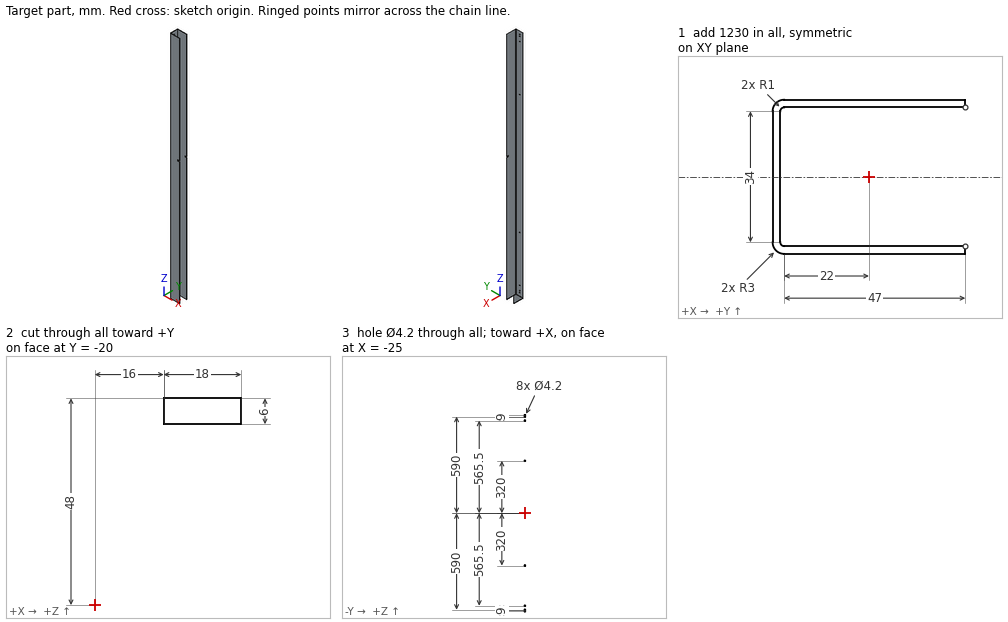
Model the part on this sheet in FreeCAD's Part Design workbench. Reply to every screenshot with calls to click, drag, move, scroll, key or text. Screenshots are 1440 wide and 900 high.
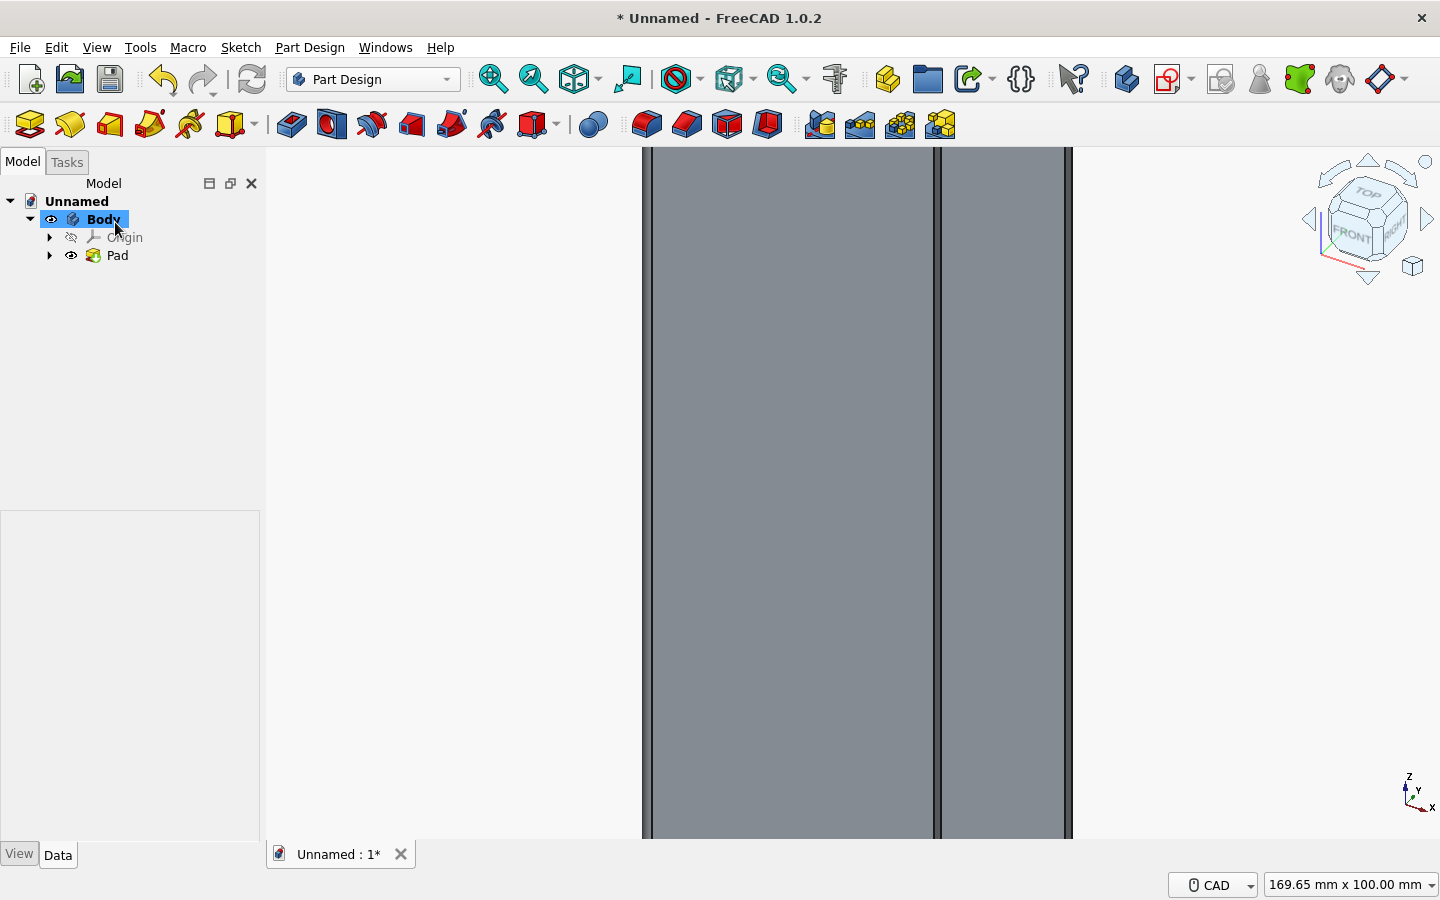
key(v)
key(f)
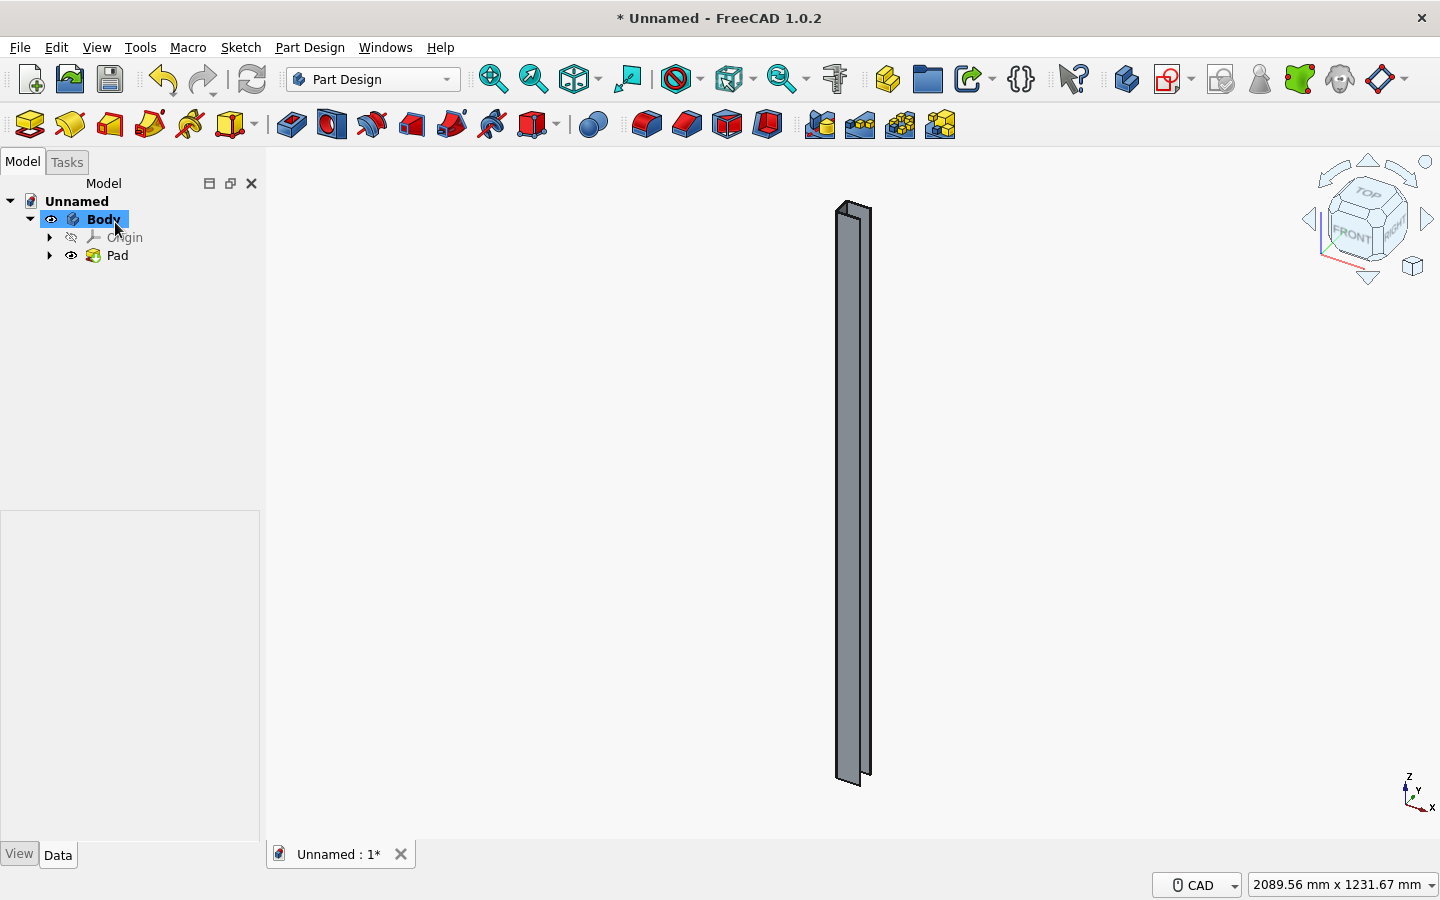
click(848, 255)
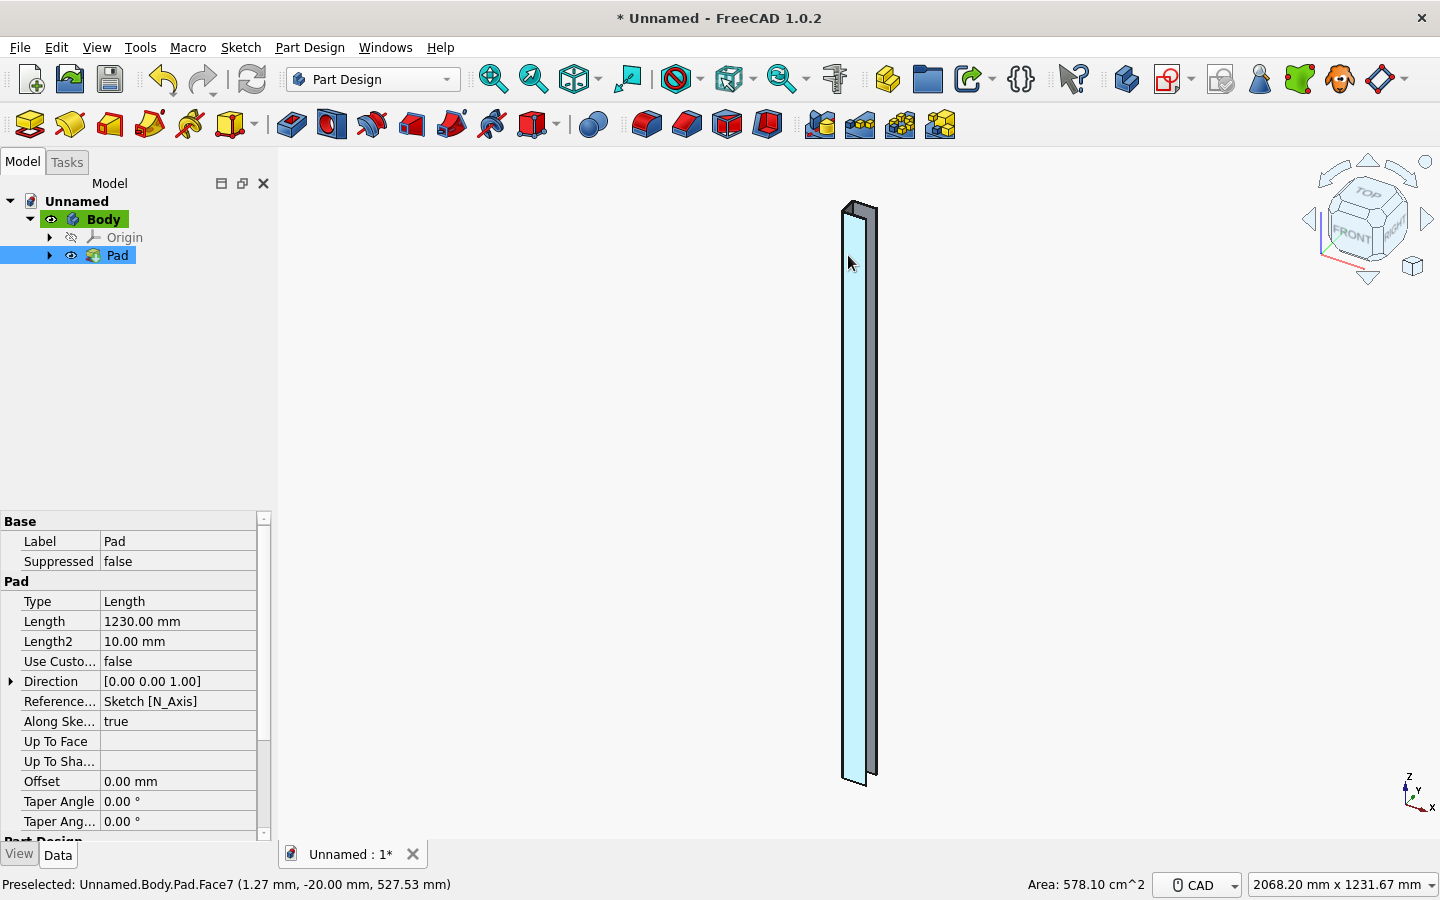
click(1168, 80)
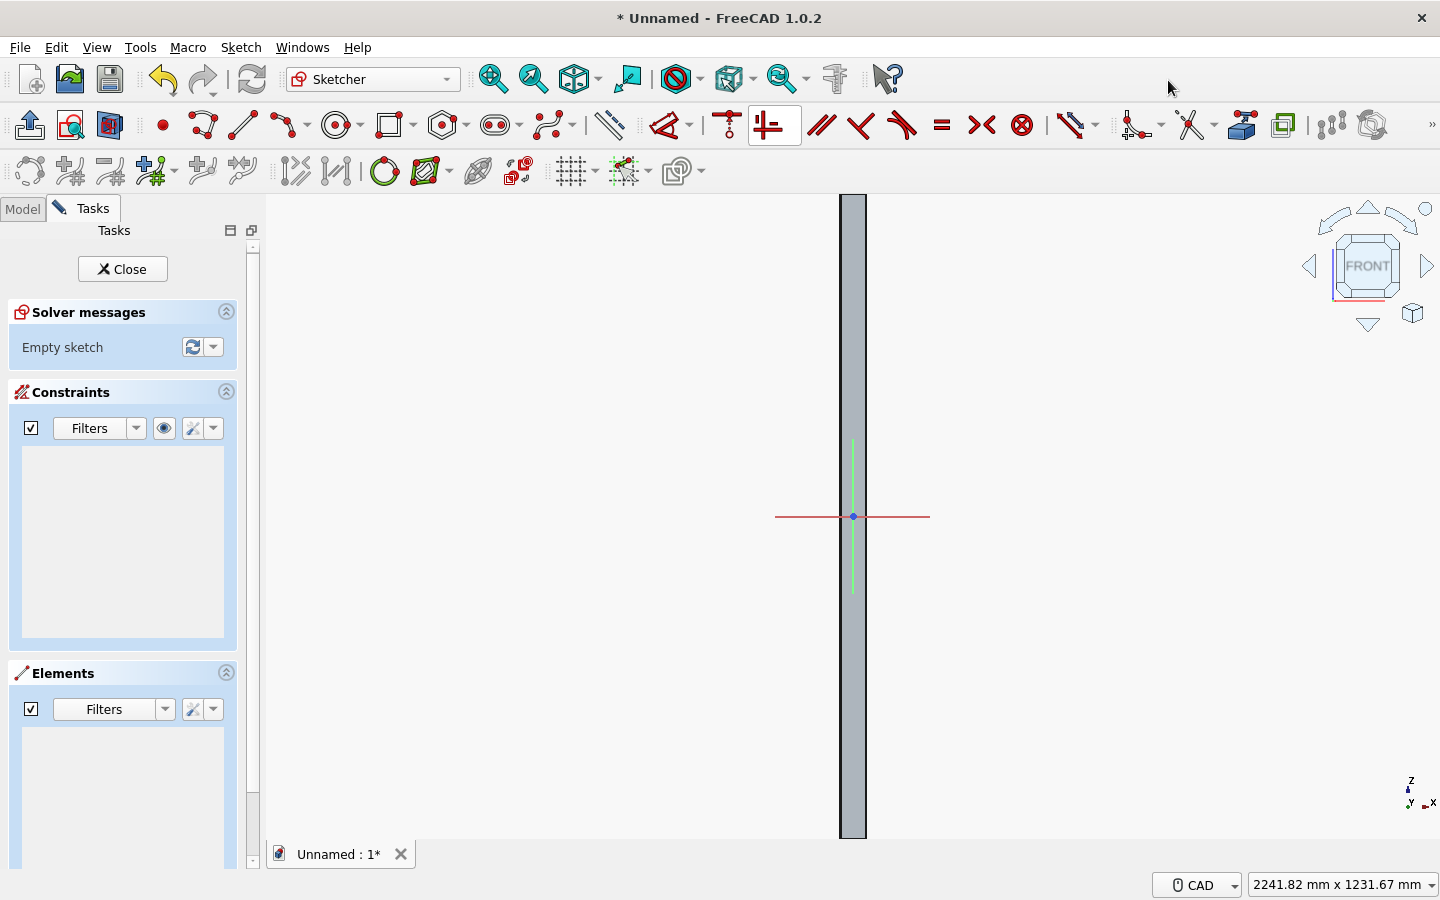
scroll(870, 492, up, 15)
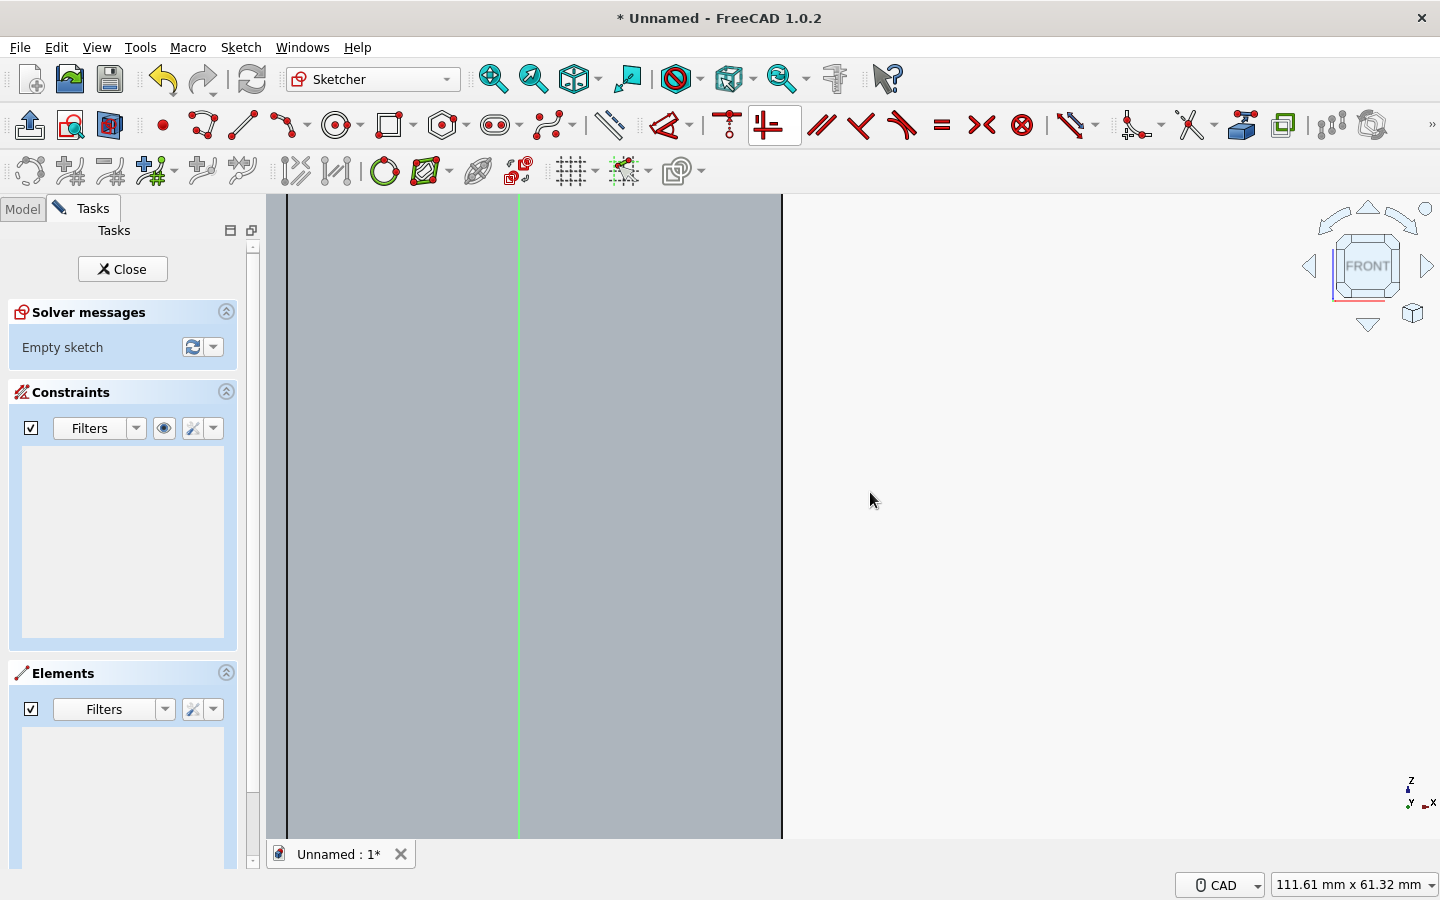
scroll(780, 496, up, 6)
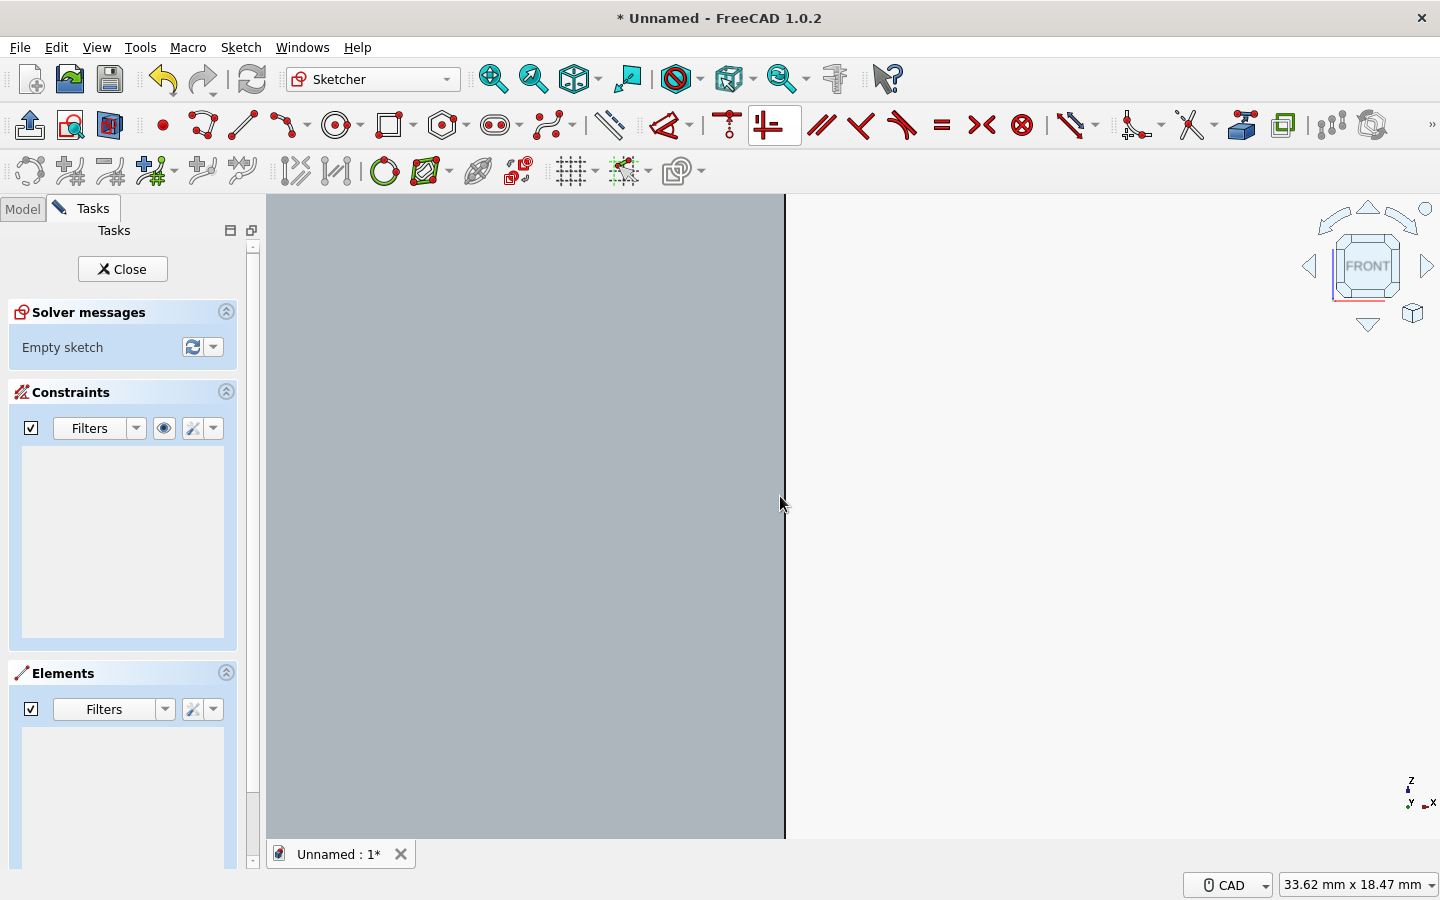
click(390, 126)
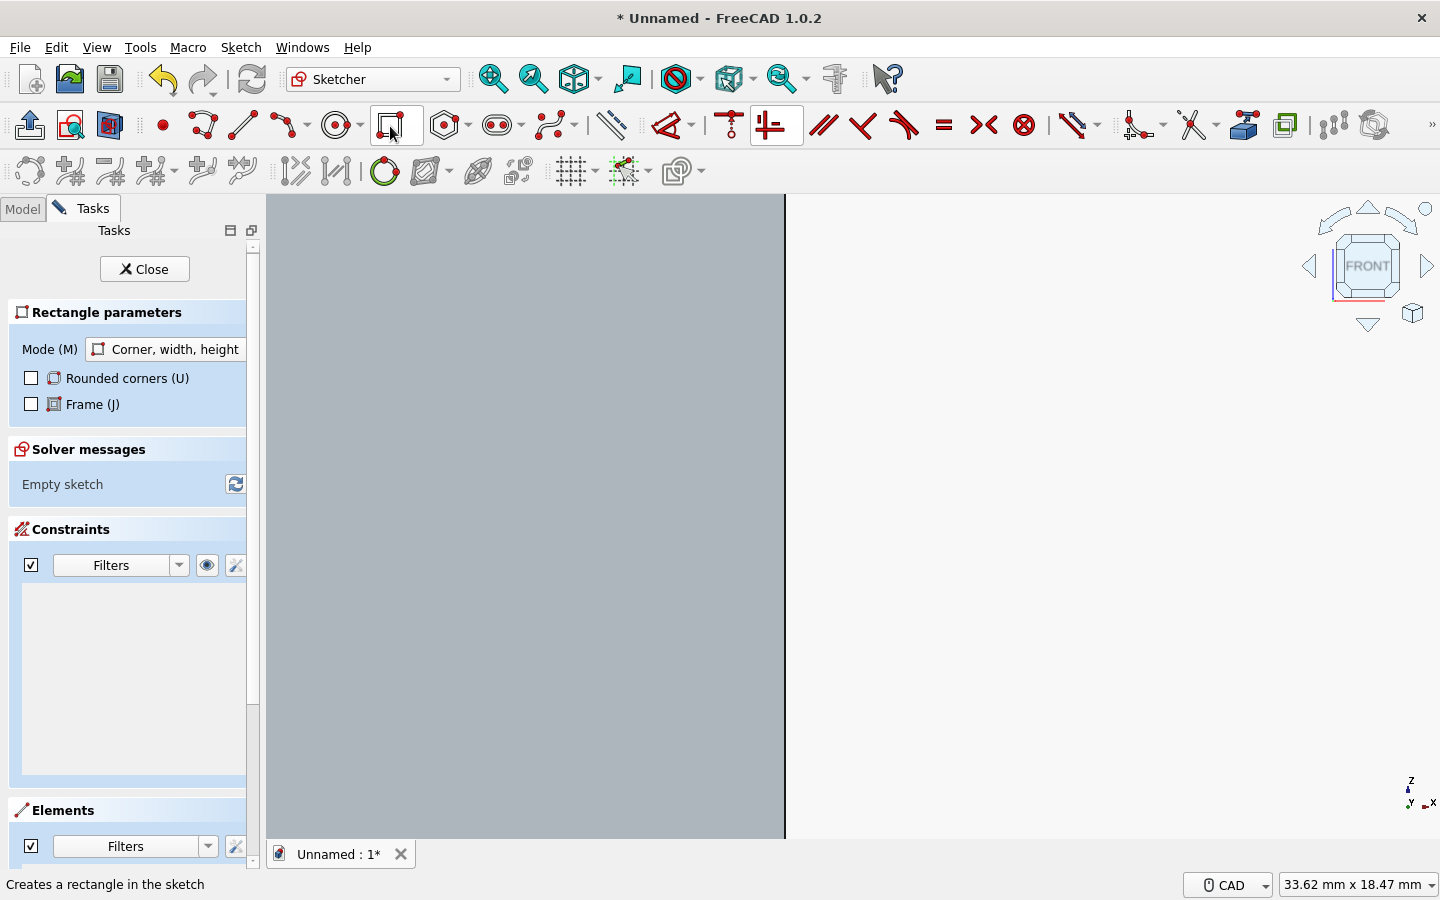
click(470, 410)
move(1099, 619)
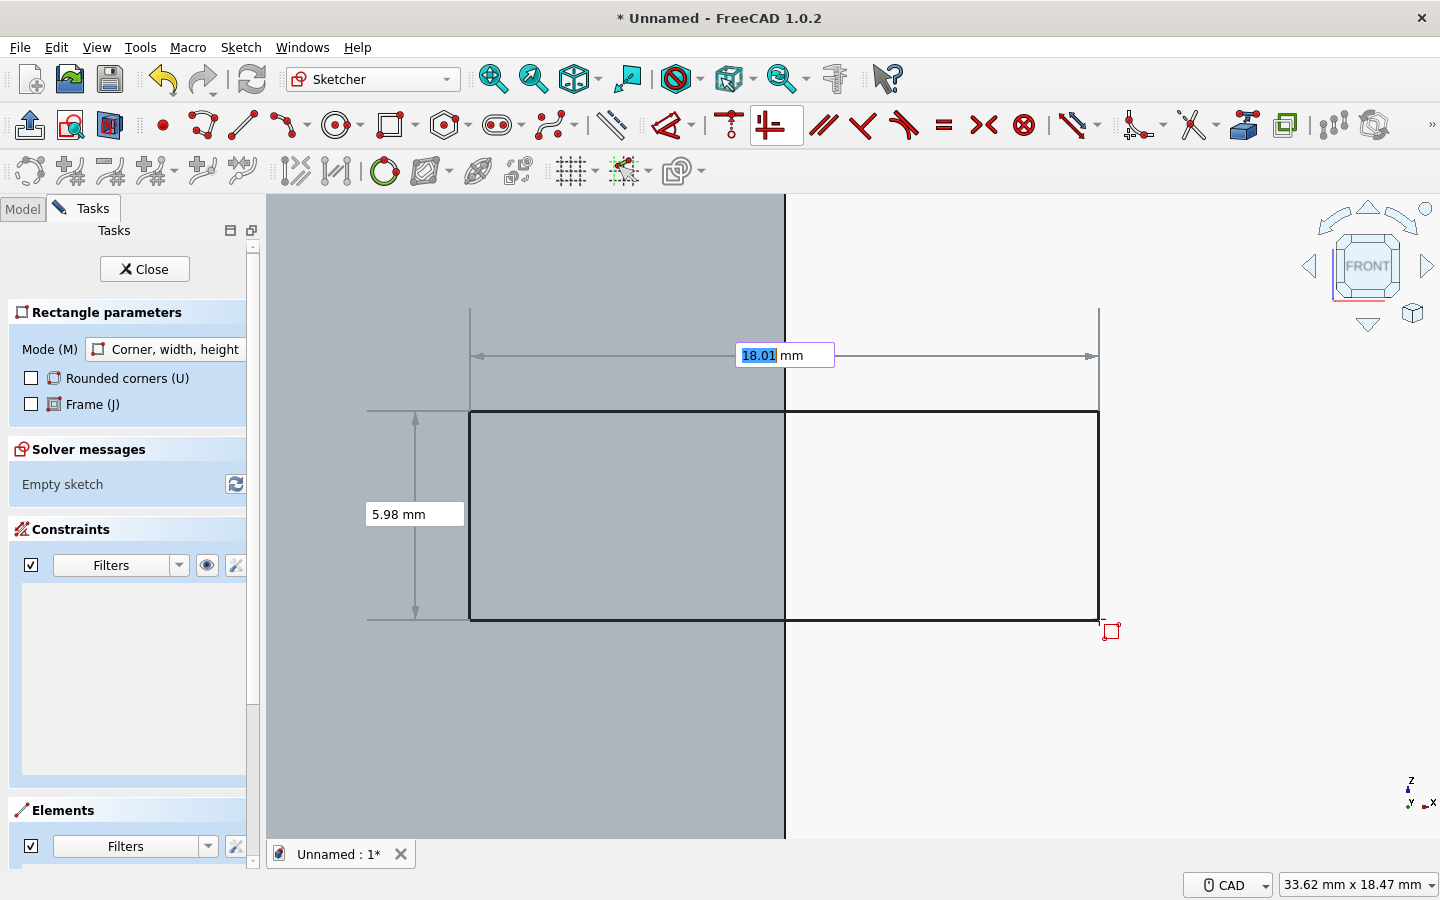
text(18)
key(Tab)
text(6)
key(Return)
key(Escape)